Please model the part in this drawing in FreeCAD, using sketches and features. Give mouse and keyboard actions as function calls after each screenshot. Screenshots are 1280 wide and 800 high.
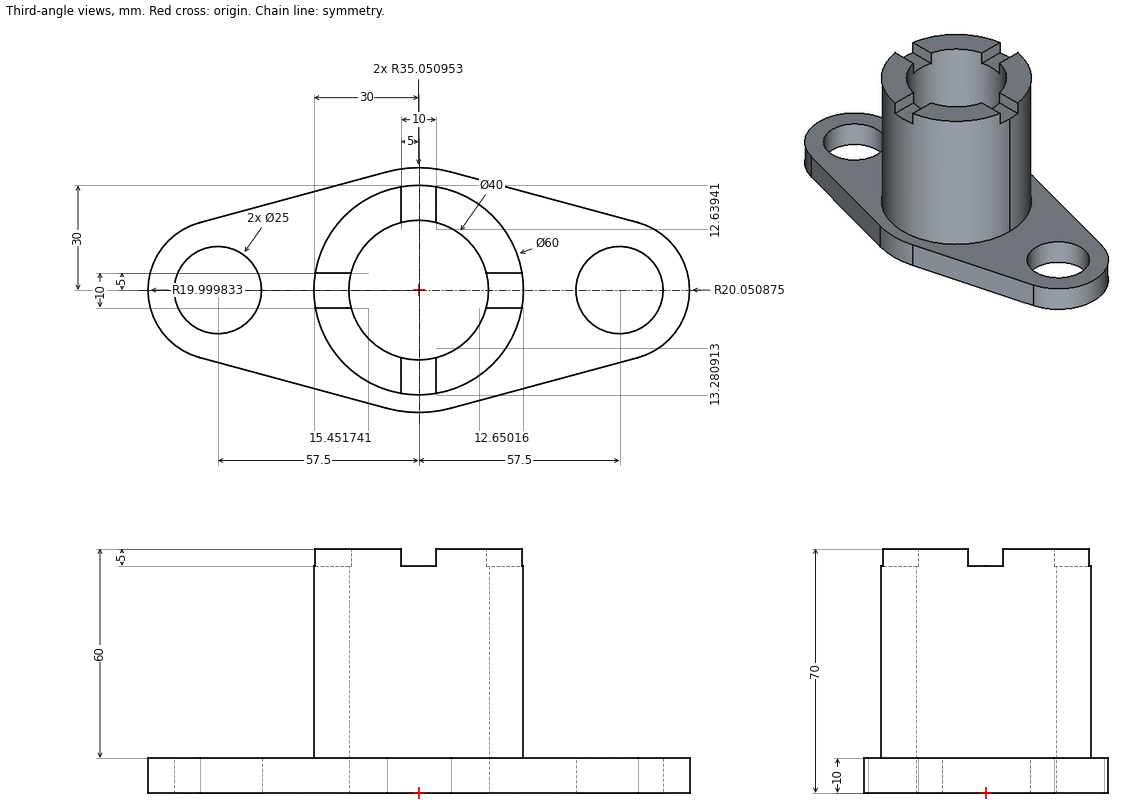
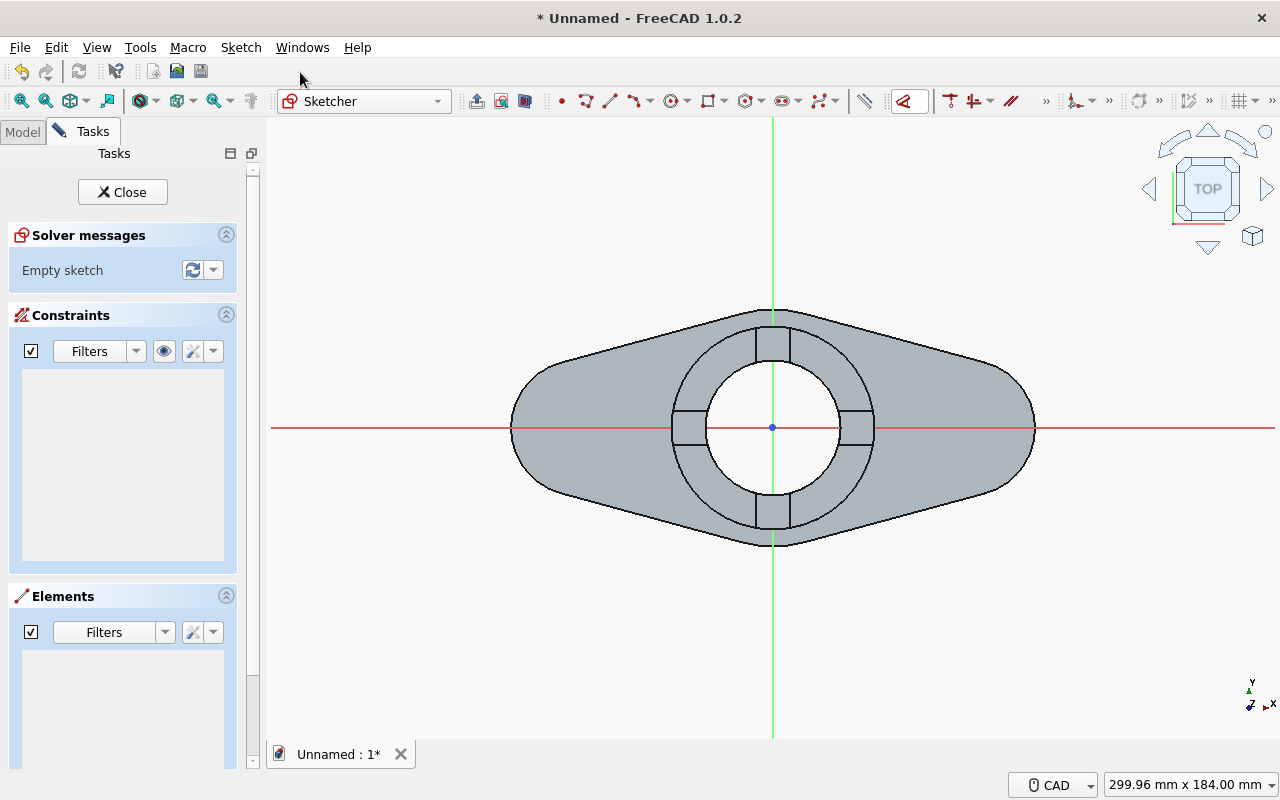
key(q)
key(s)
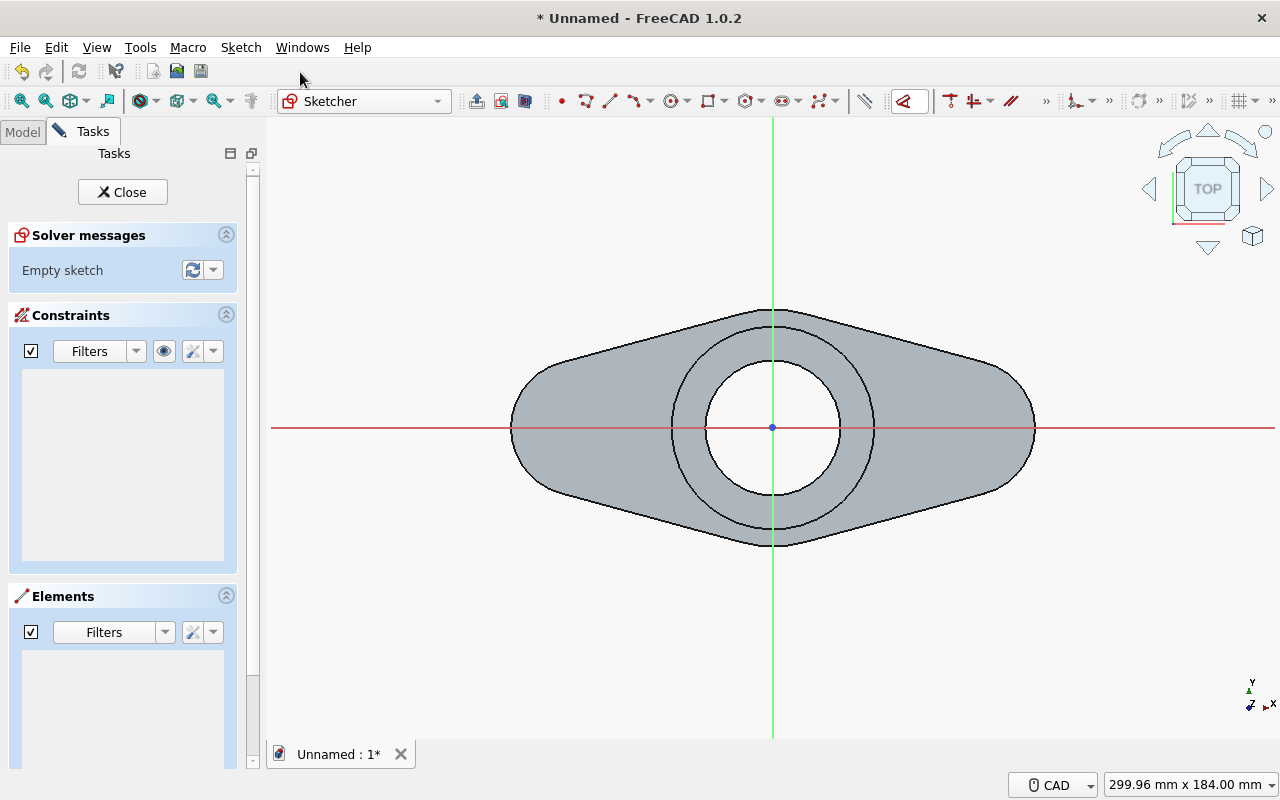
click(672, 102)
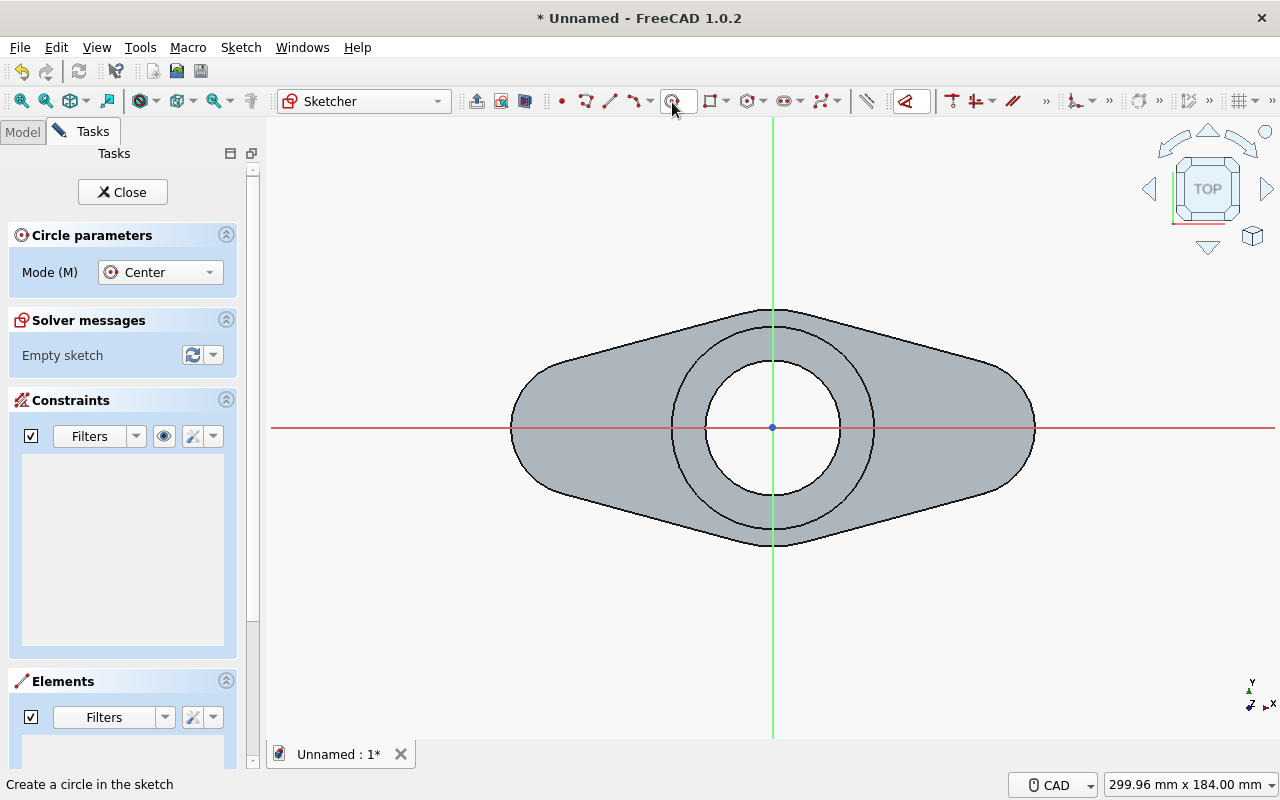
click(579, 428)
move(608, 398)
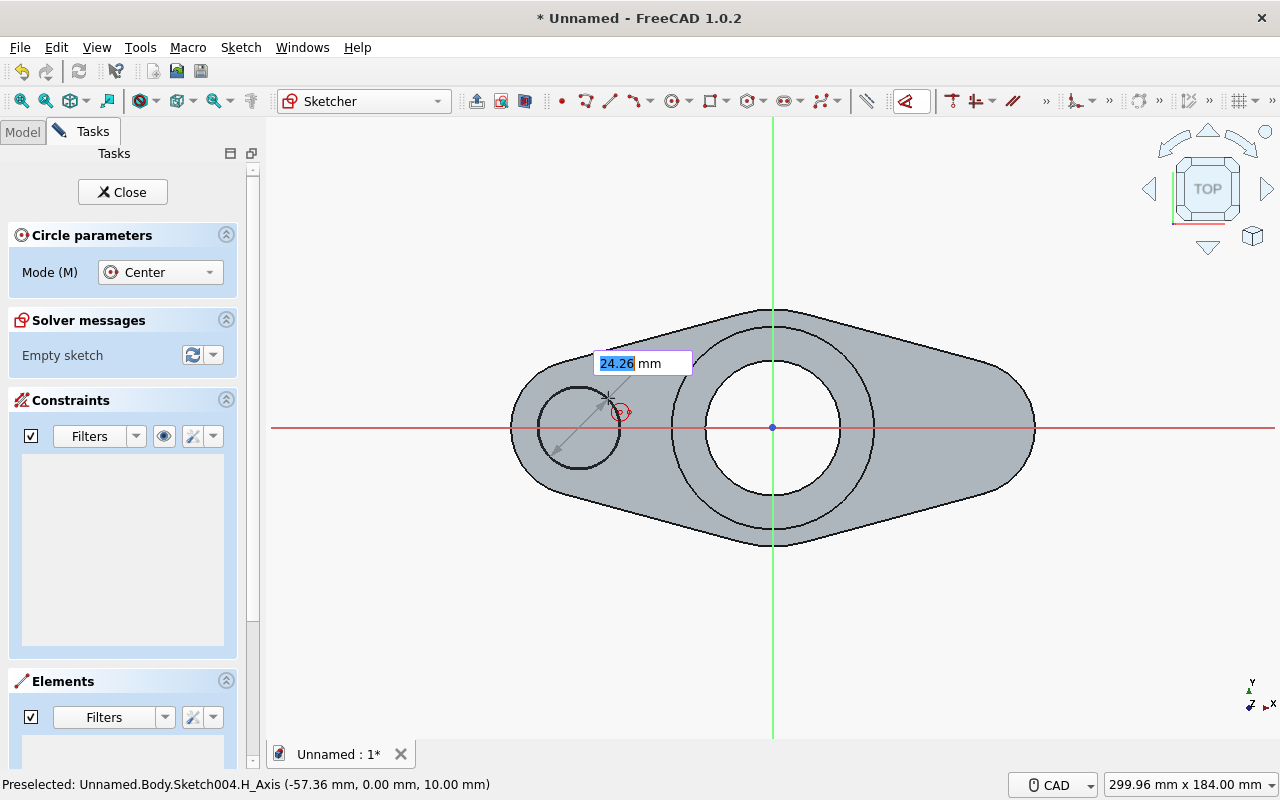
text(25)
key(Return)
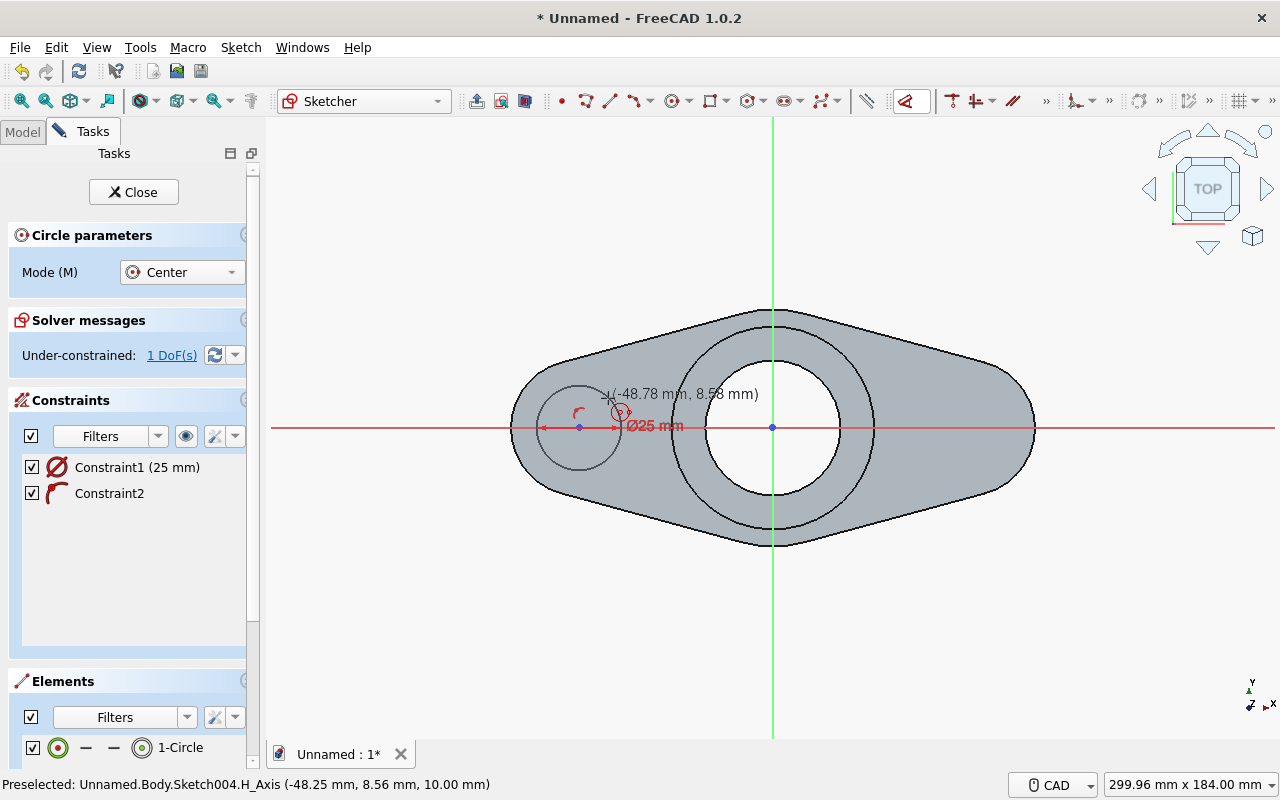
click(967, 428)
move(997, 398)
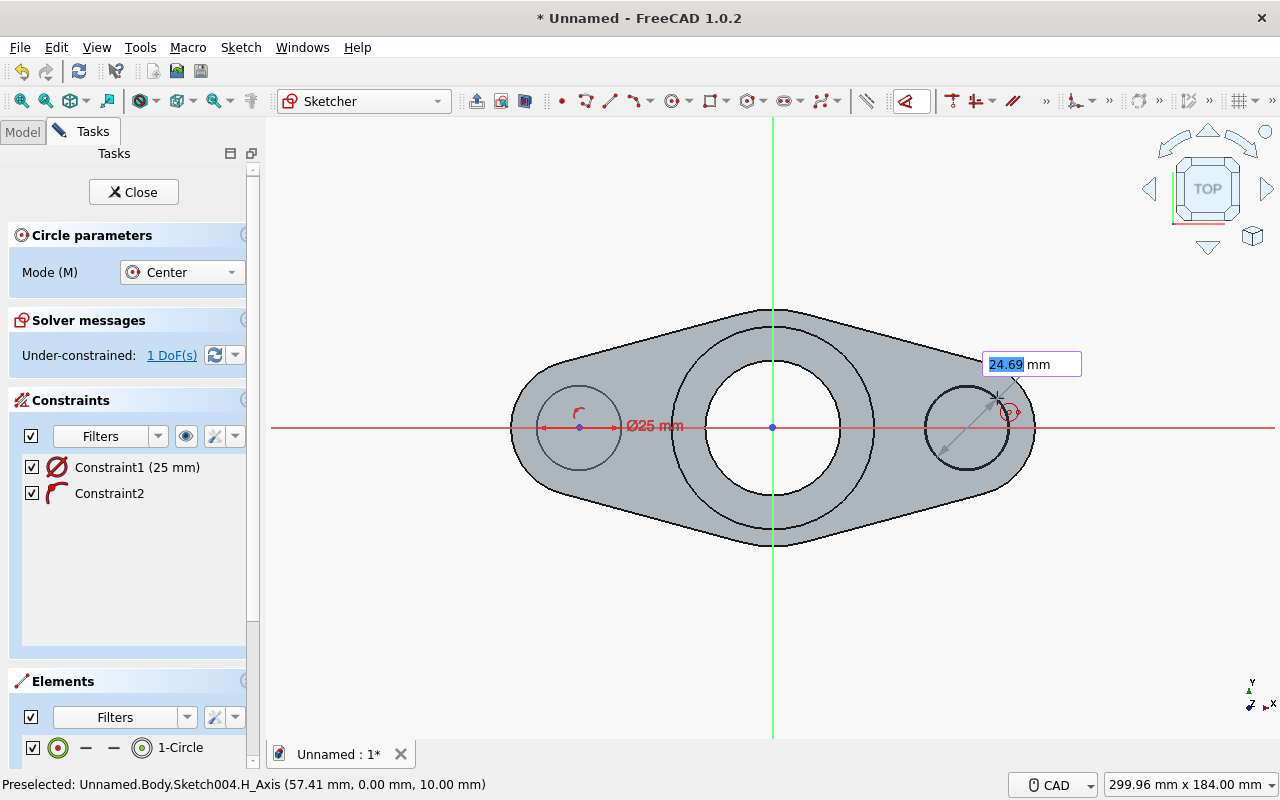
text(25)
key(Return)
key(Escape)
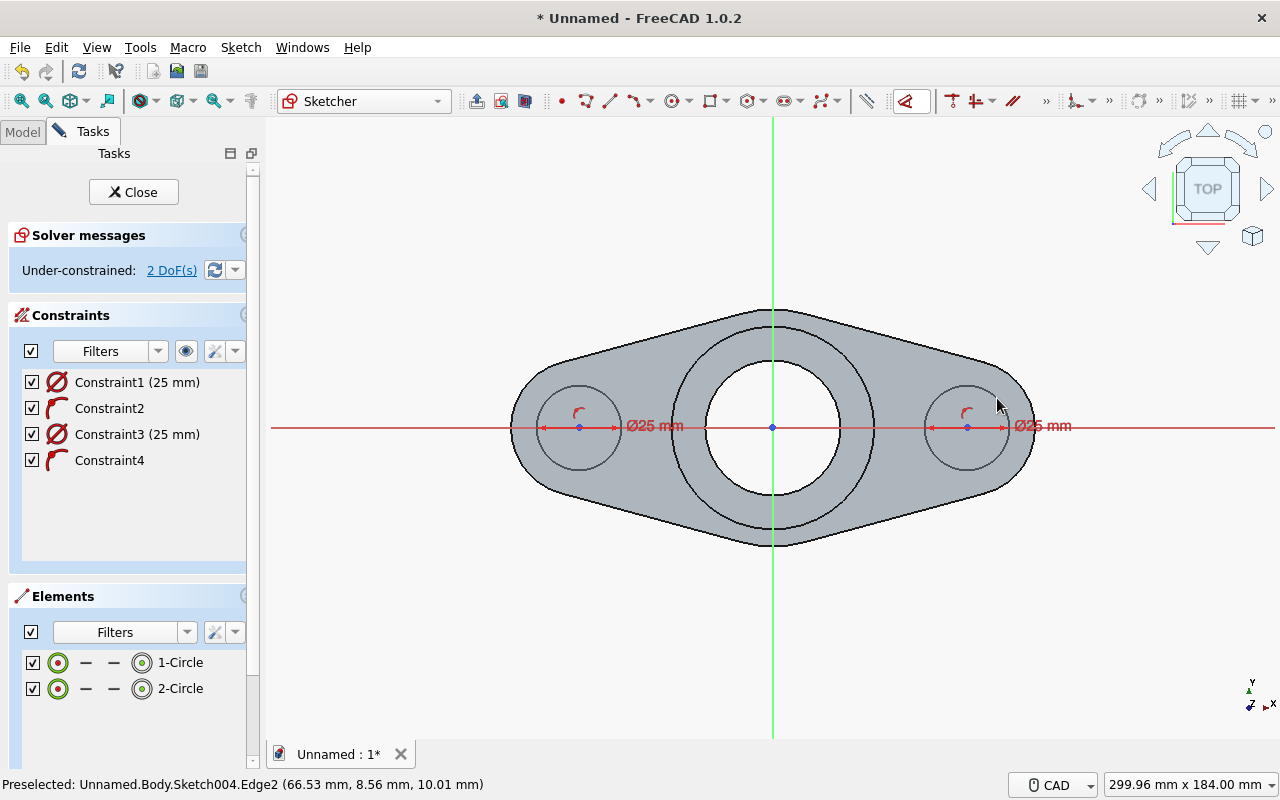
click(579, 428)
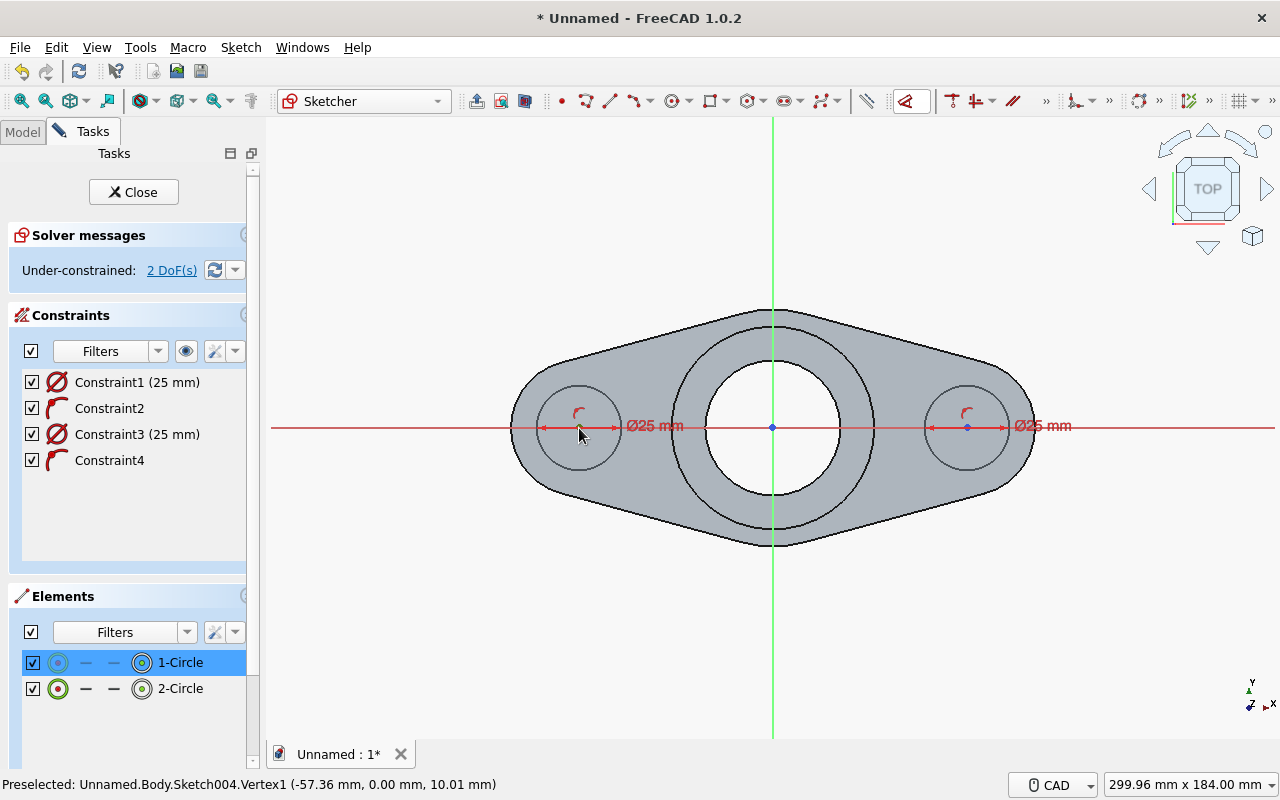
key(l)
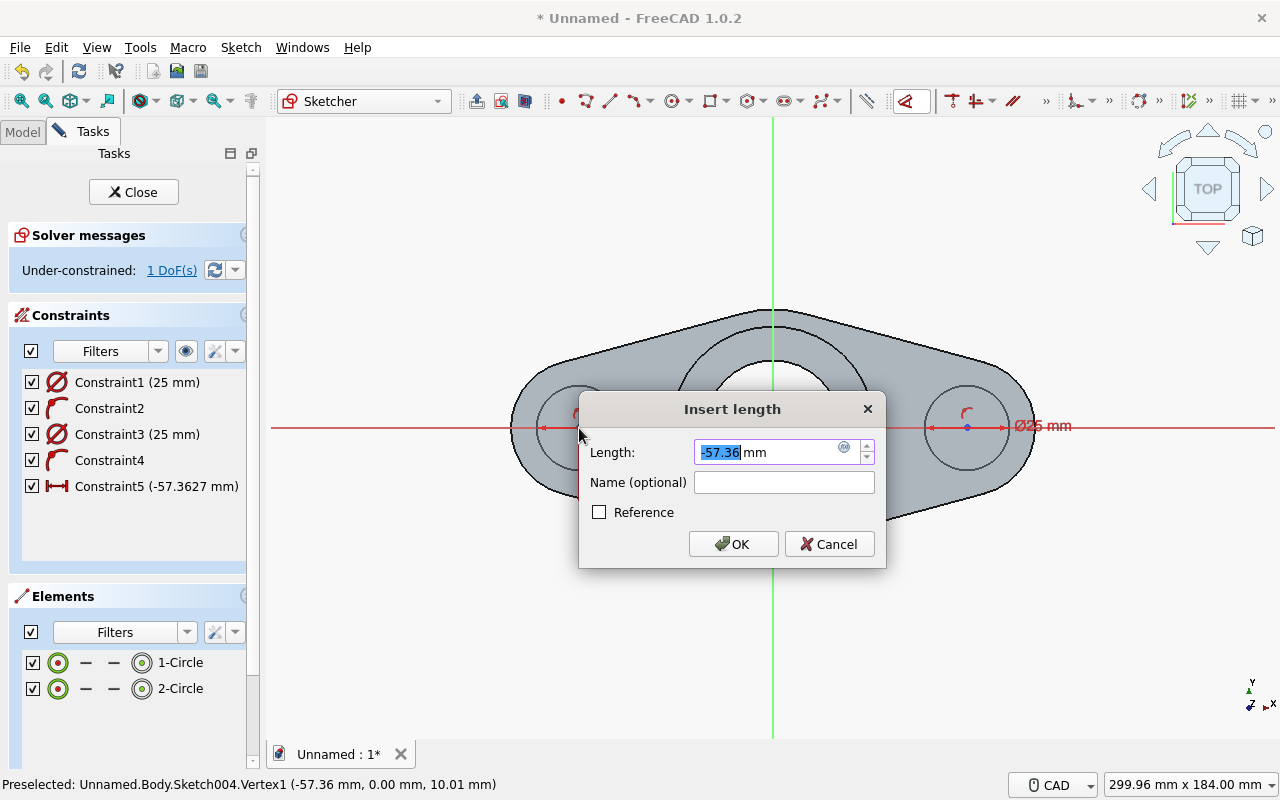
text(-57.5)
key(Return)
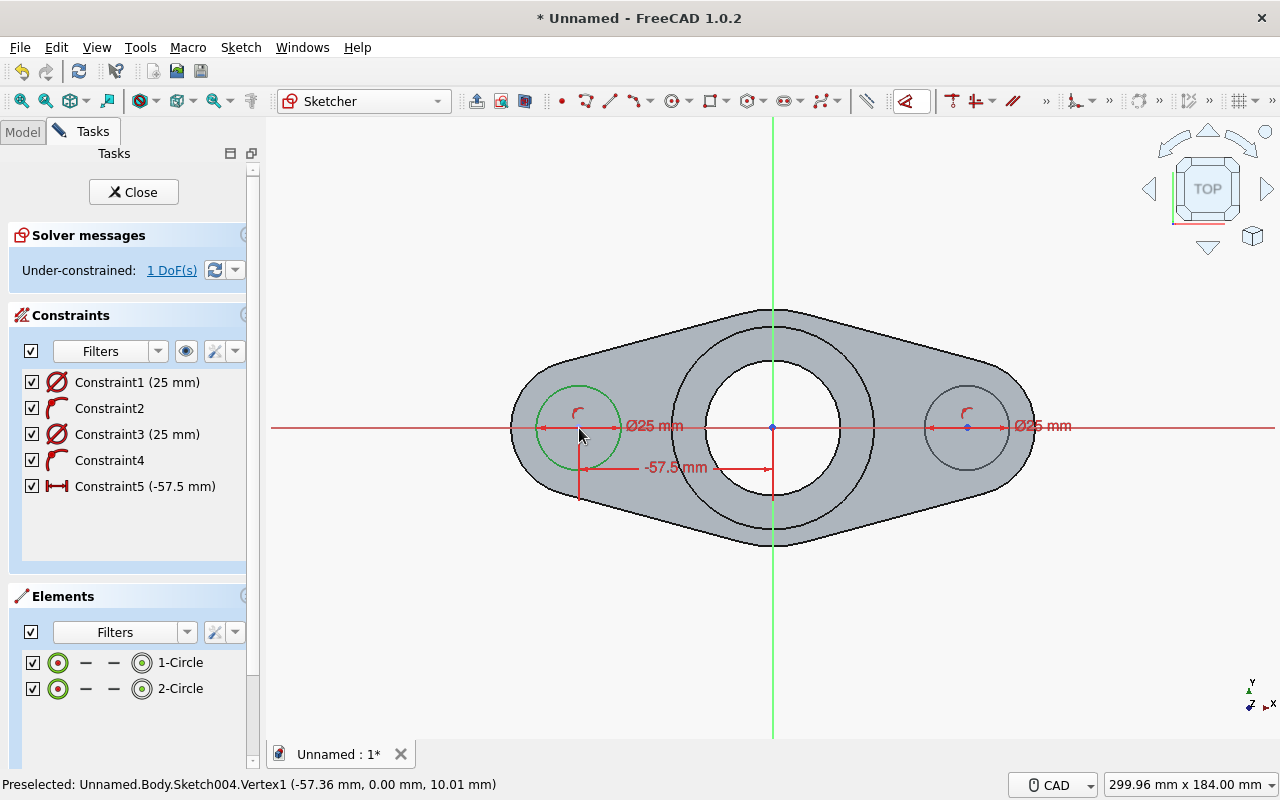
click(967, 428)